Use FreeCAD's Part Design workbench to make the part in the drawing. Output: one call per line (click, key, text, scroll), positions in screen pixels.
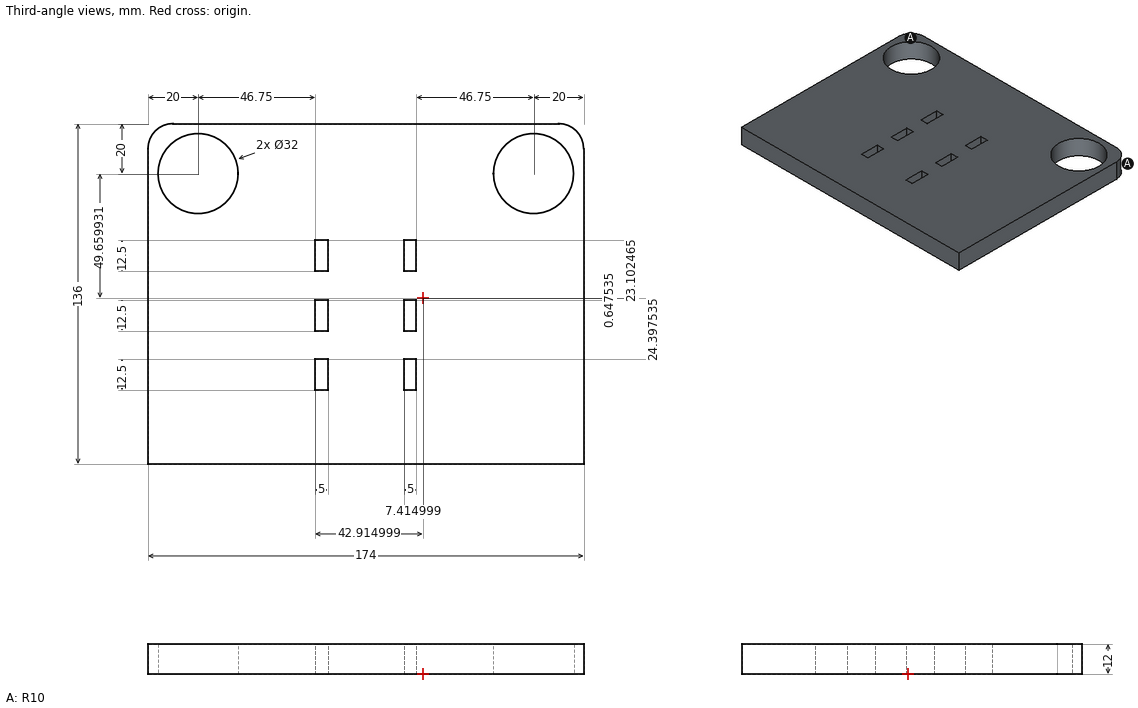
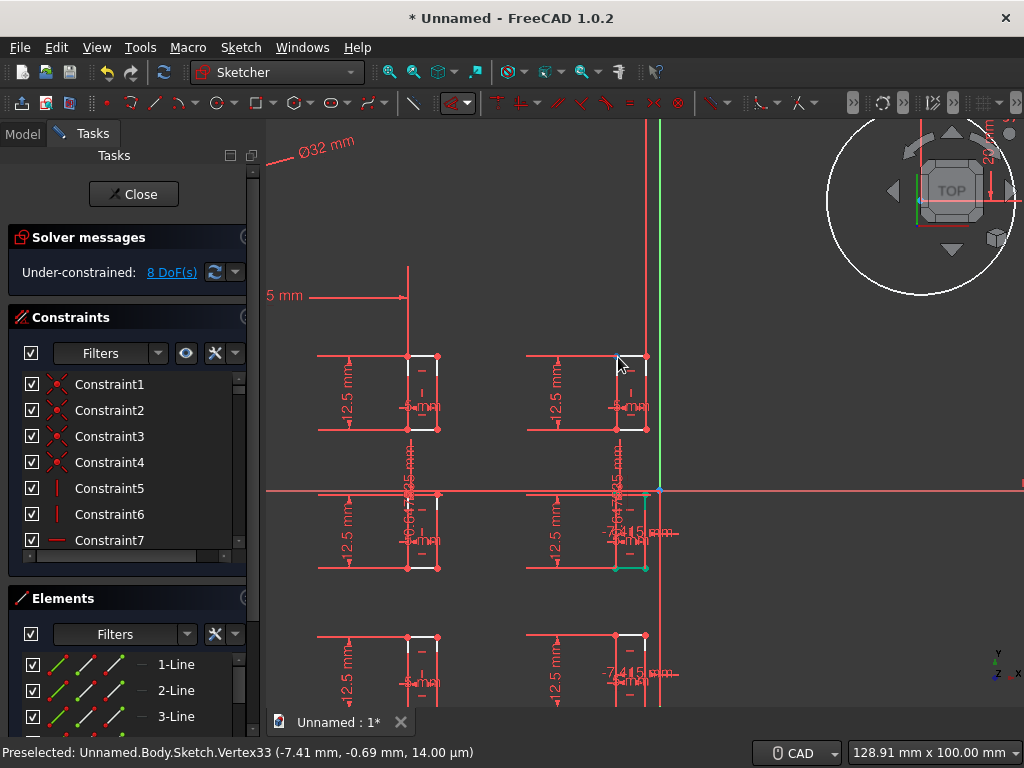
click(617, 356)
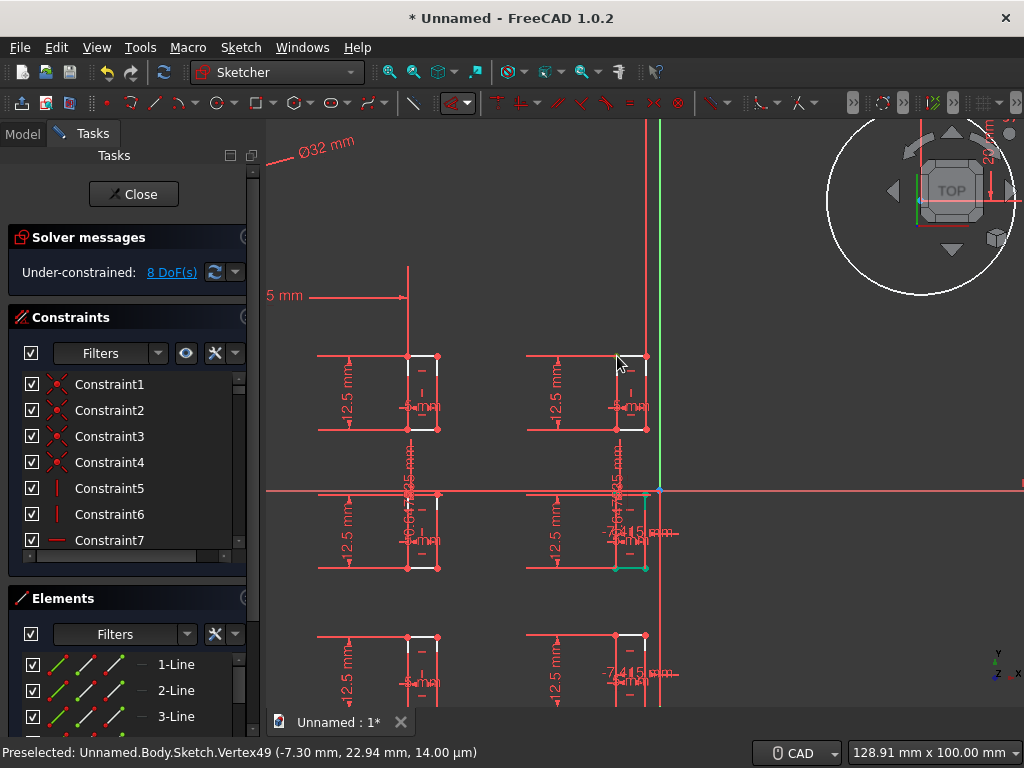
click(470, 104)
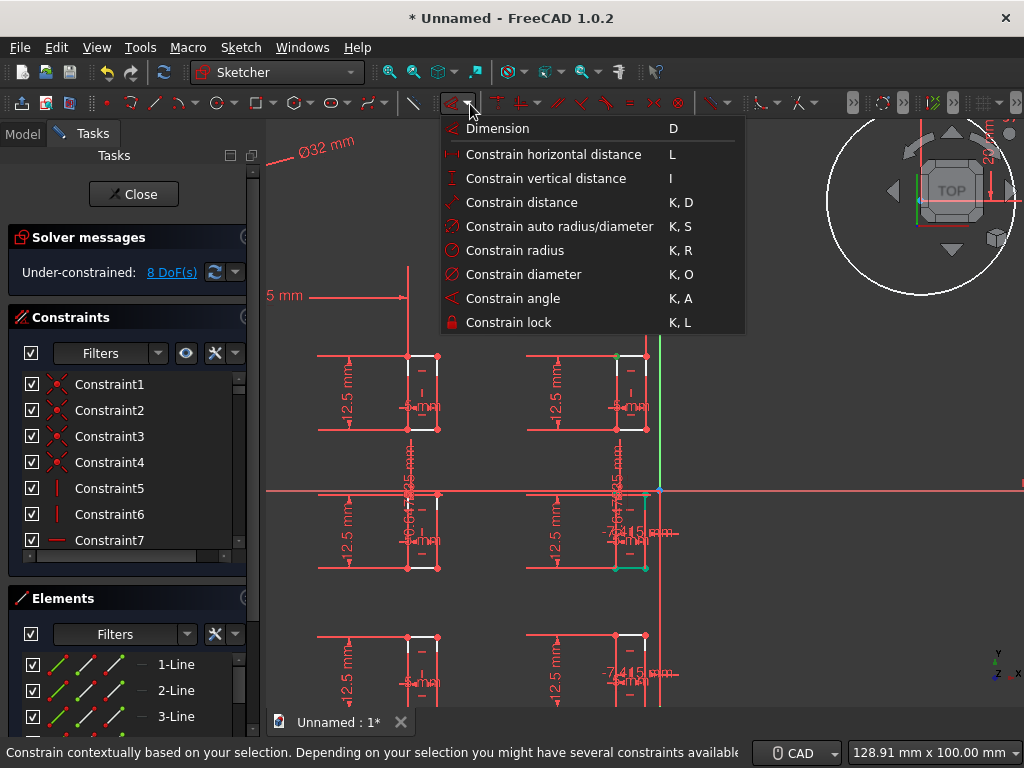
click(593, 154)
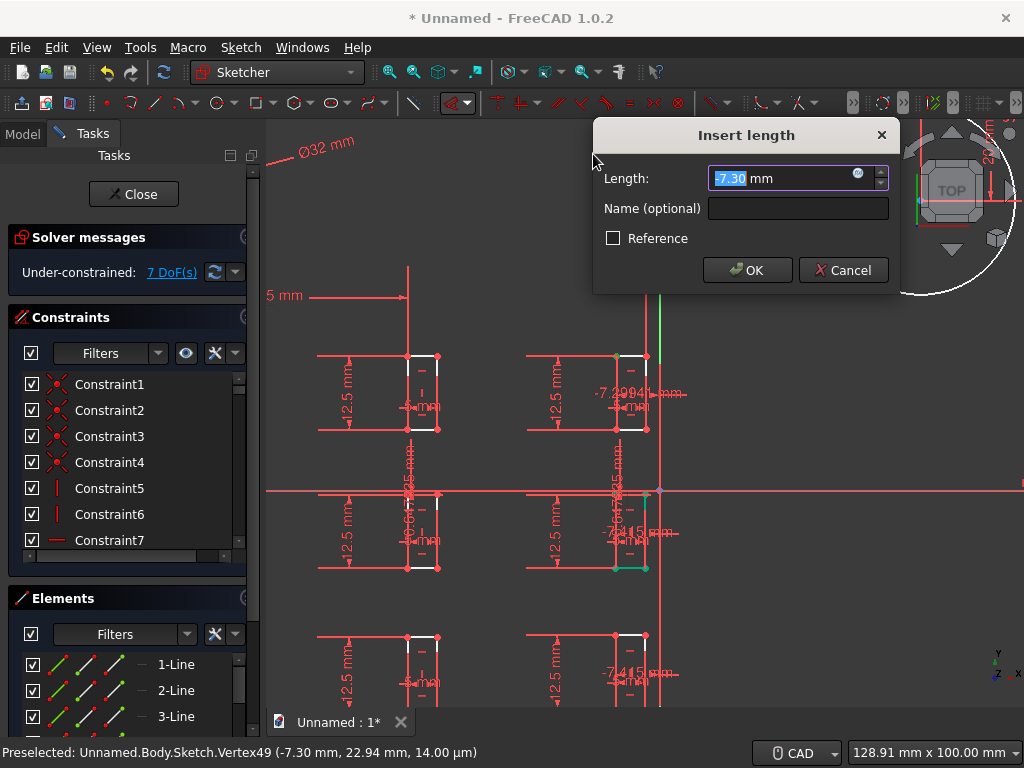
text(-7.414999)
key(Return)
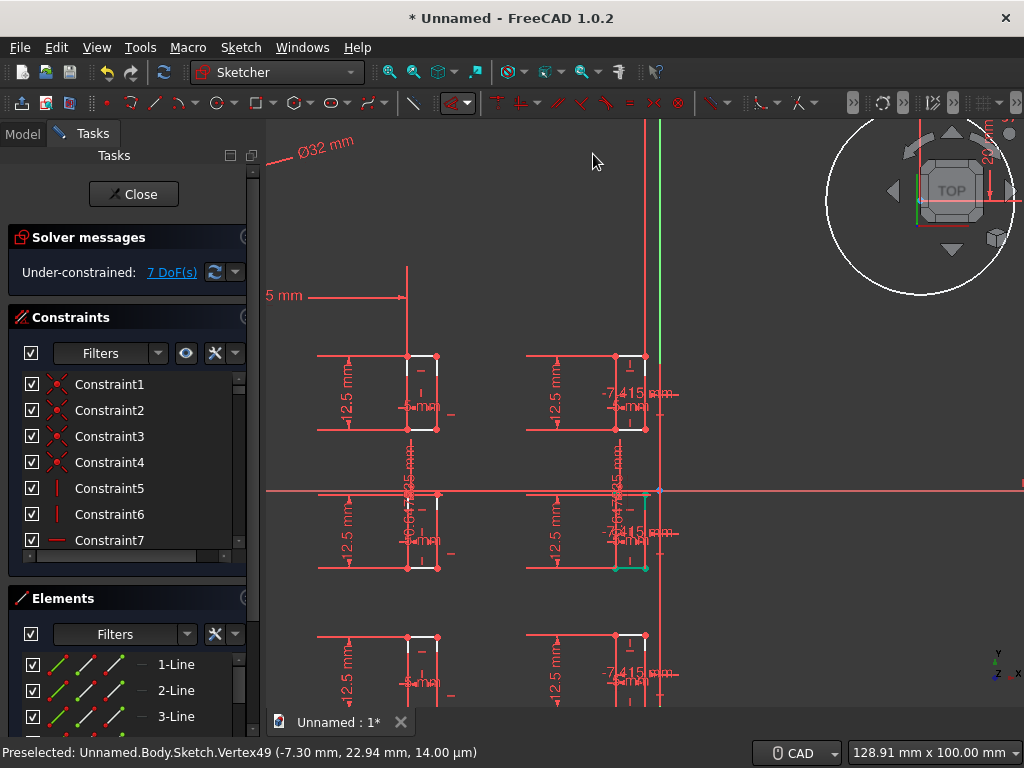
scroll(606, 373, down, 5)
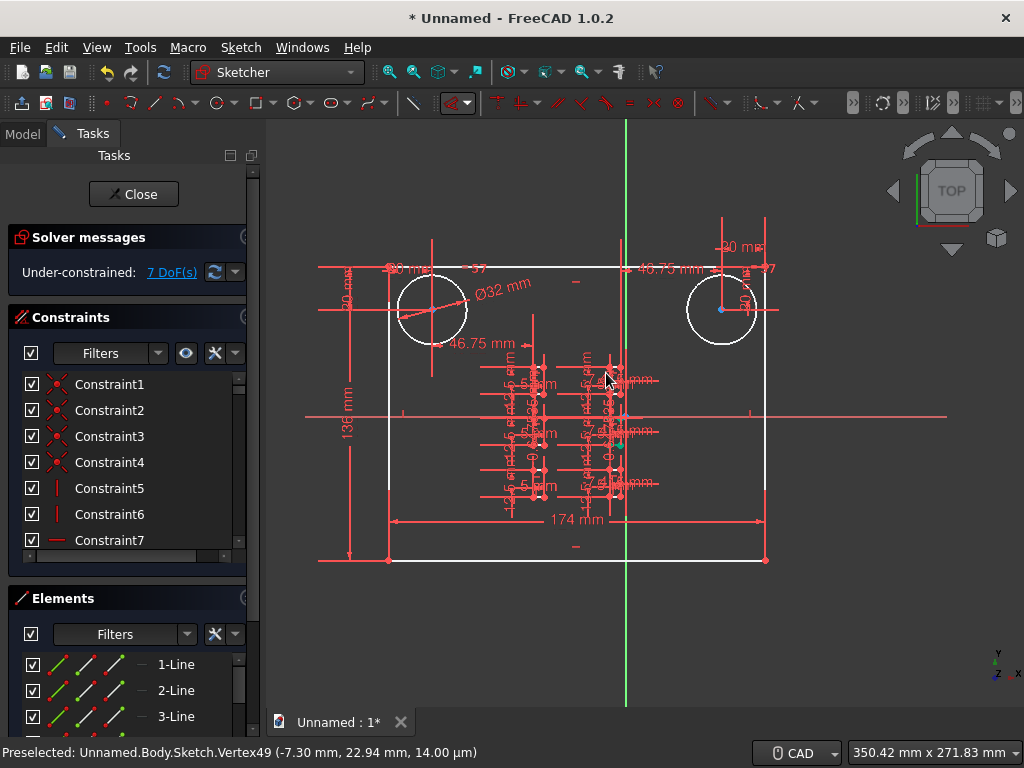
click(432, 310)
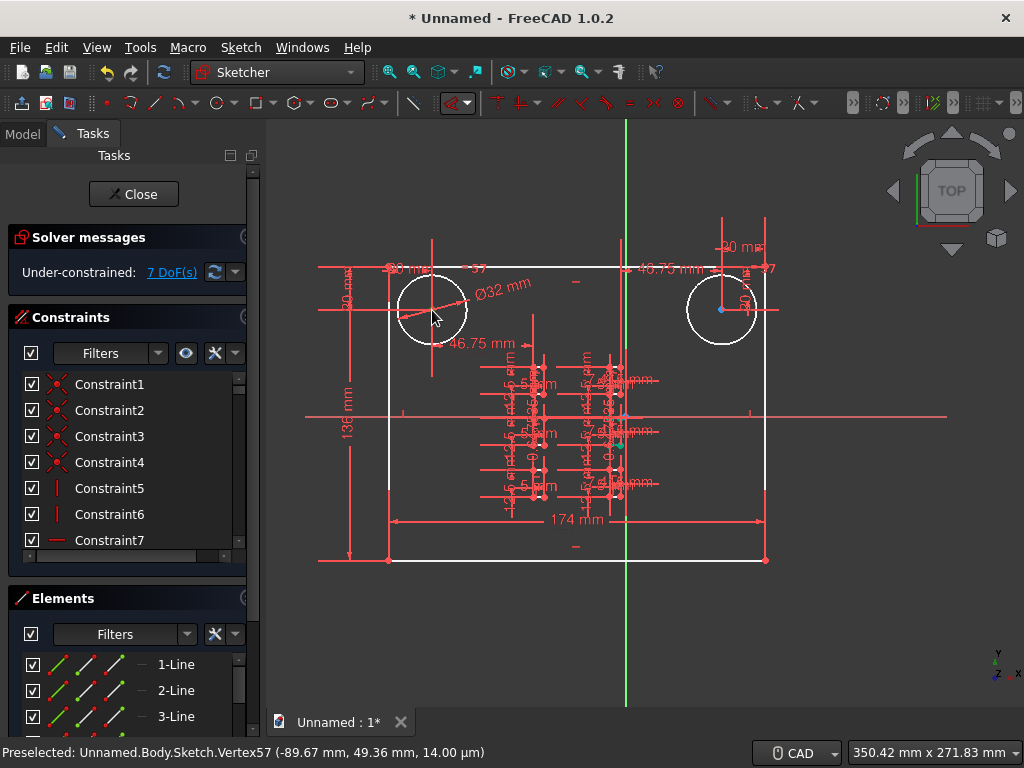
key(i)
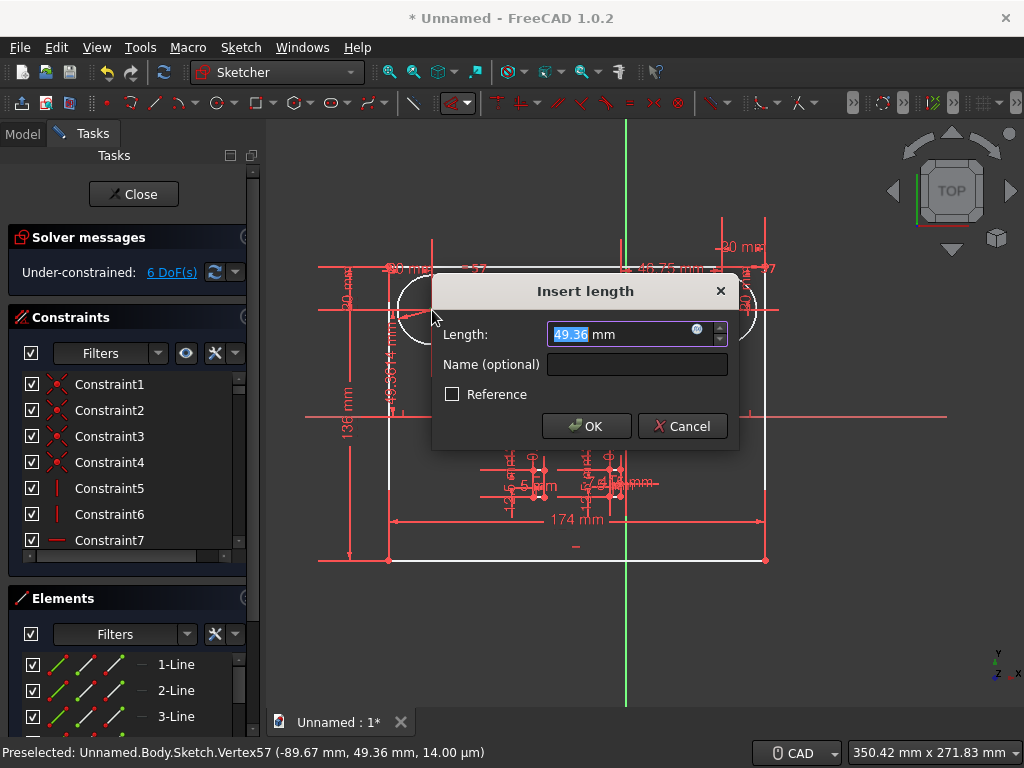
text(49.659931)
key(Return)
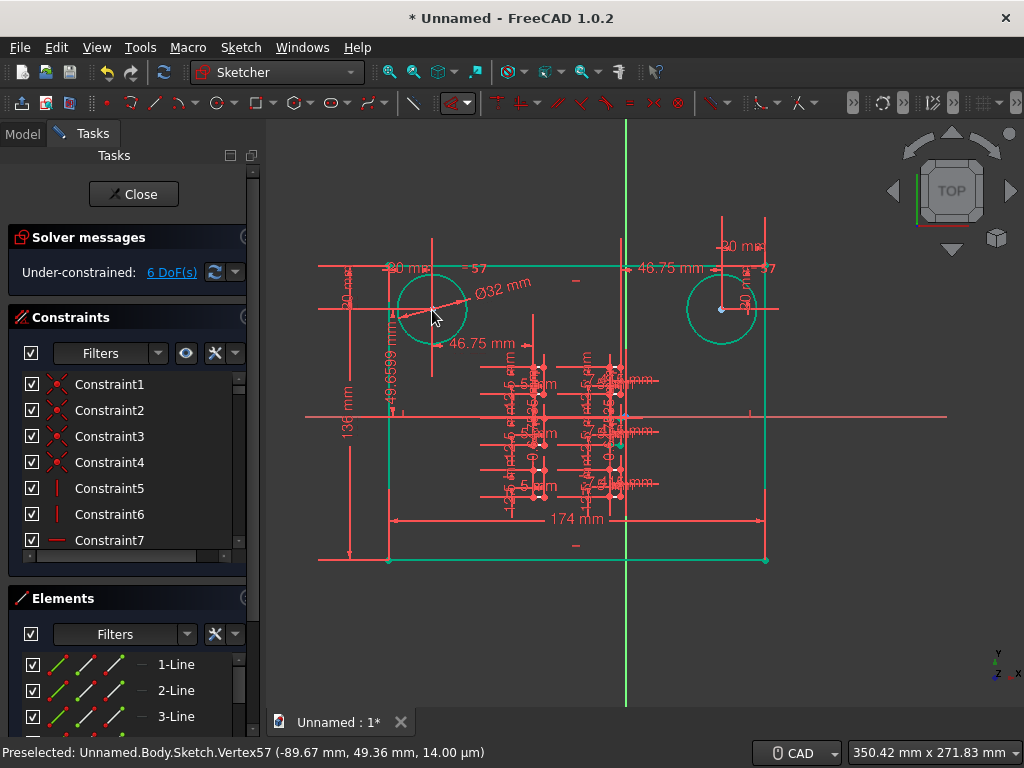
click(533, 470)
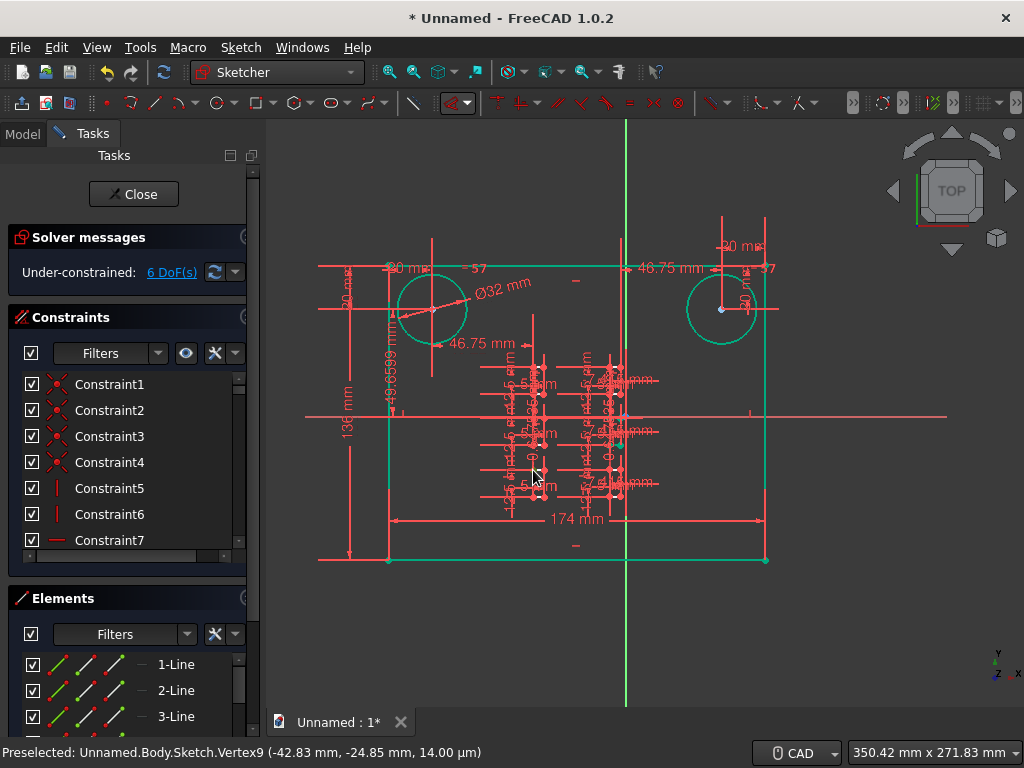
click(470, 104)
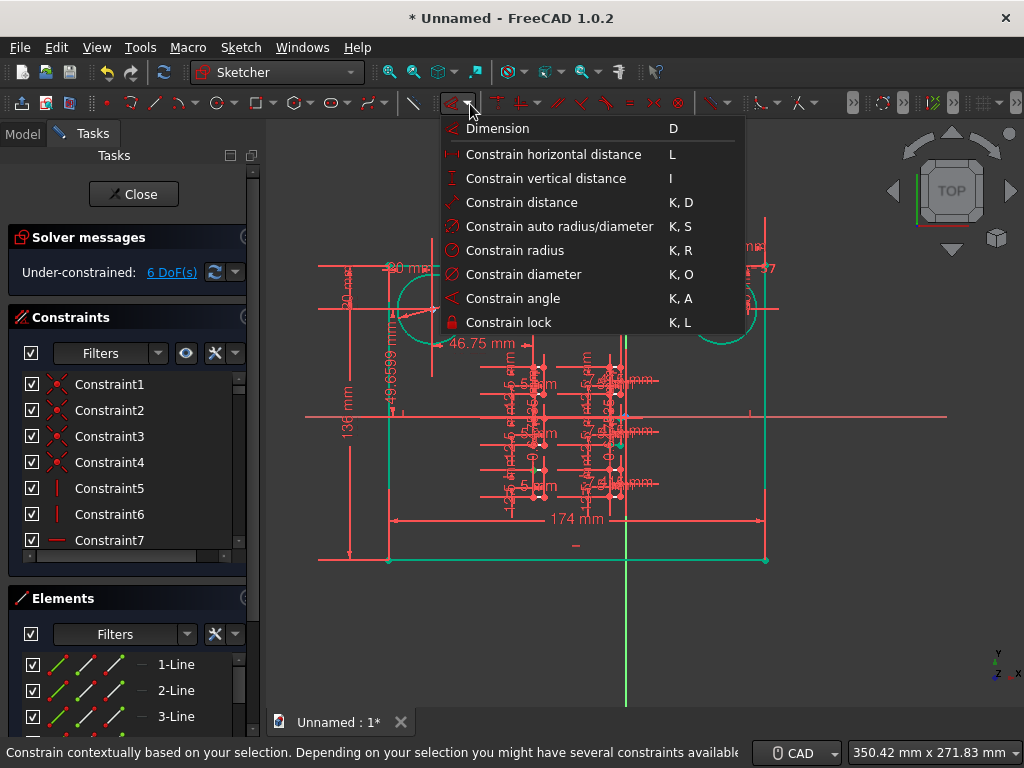
click(593, 154)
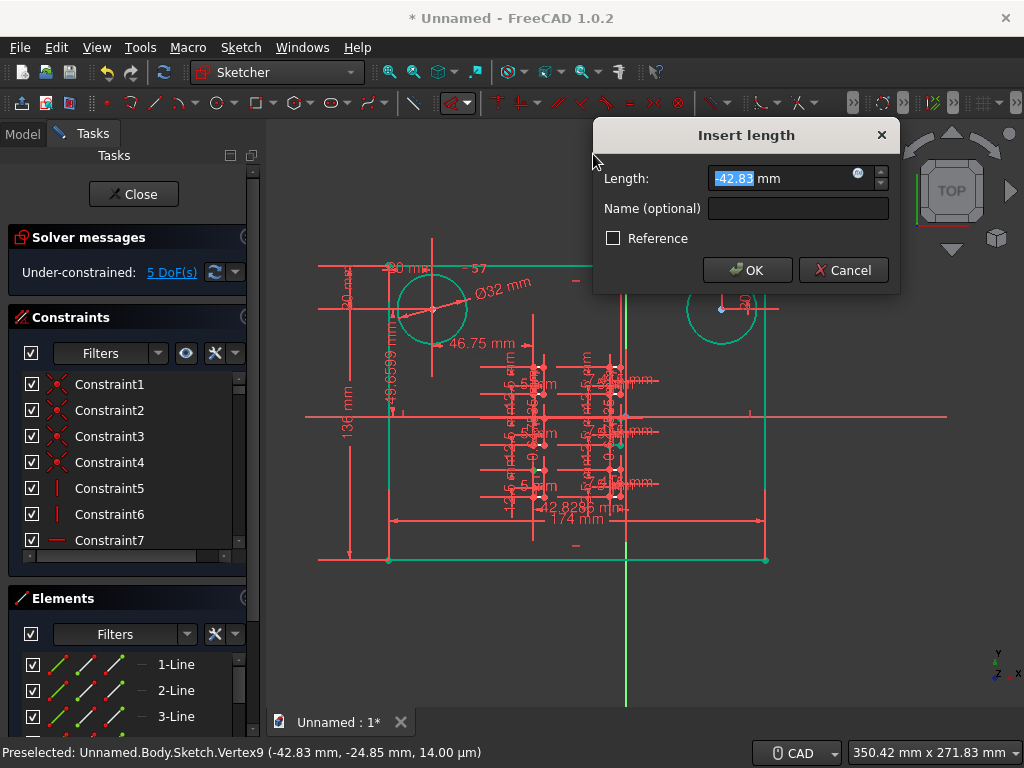
text(-42.914999)
key(Return)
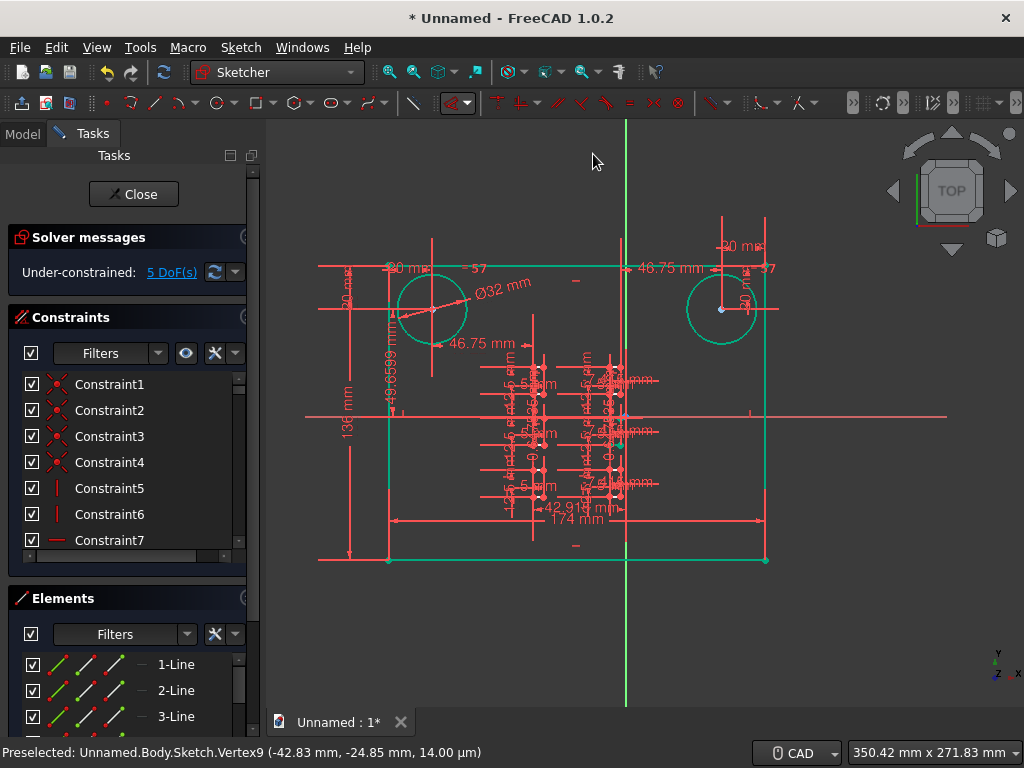
click(533, 470)